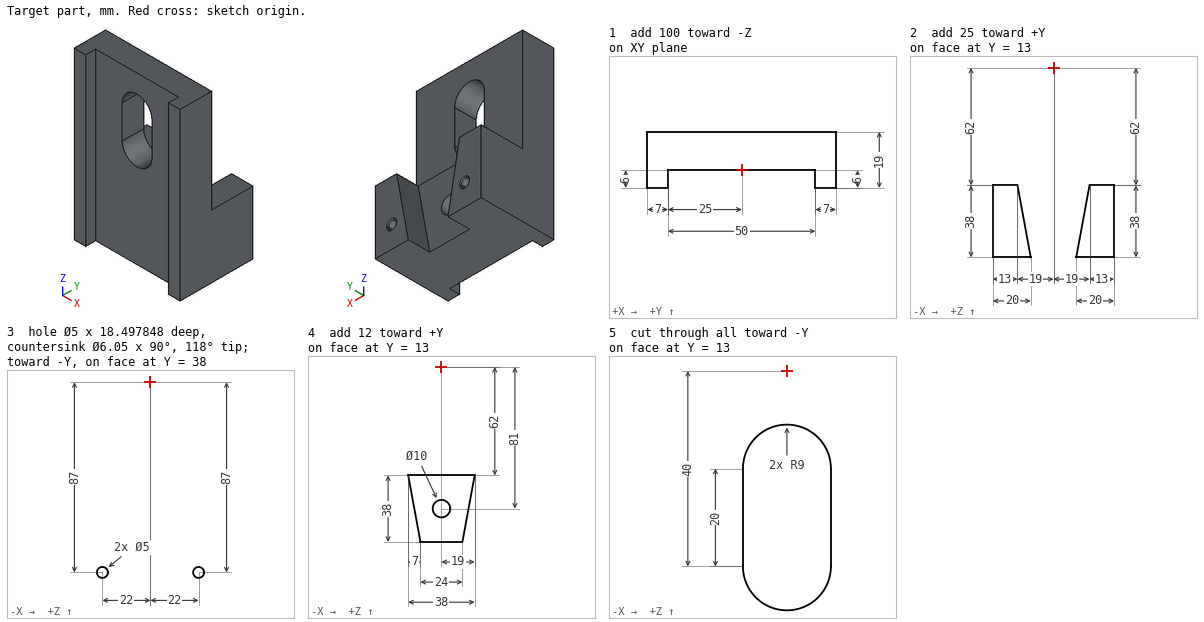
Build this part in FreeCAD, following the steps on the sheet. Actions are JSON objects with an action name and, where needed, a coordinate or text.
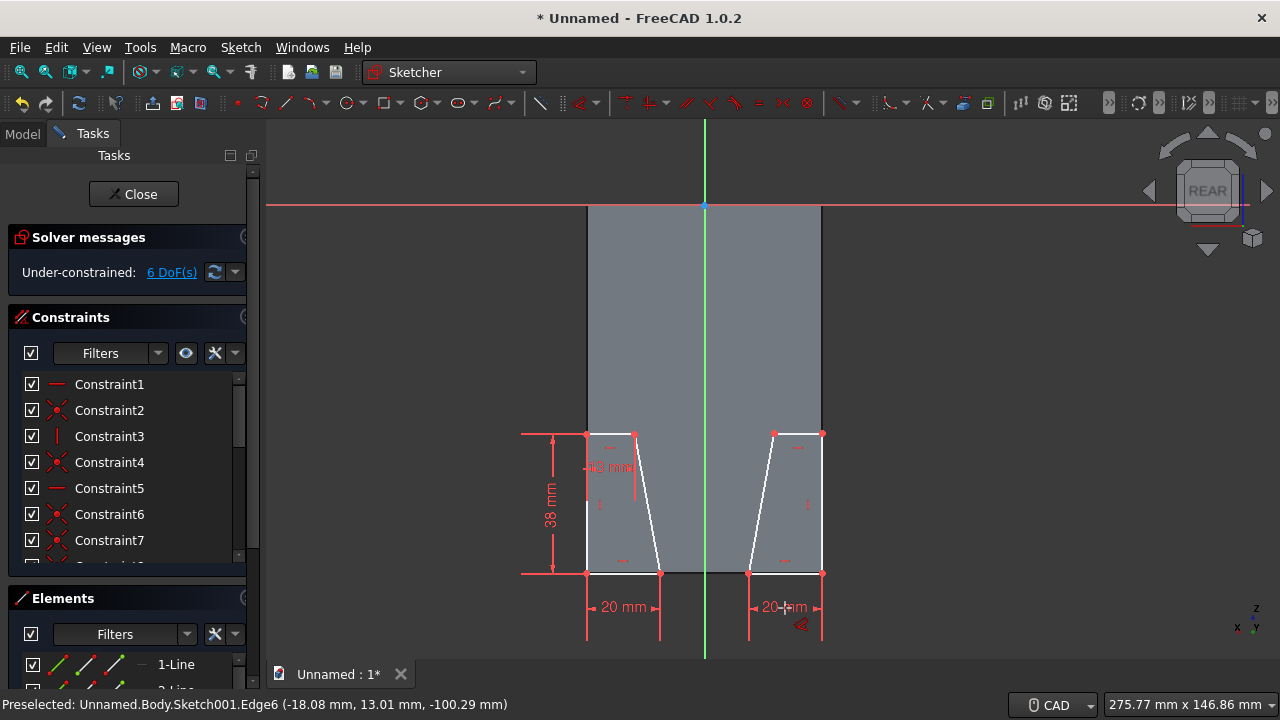
{"action": "left_click", "coordinate": [822, 532]}
{"action": "left_click", "coordinate": [856, 504]}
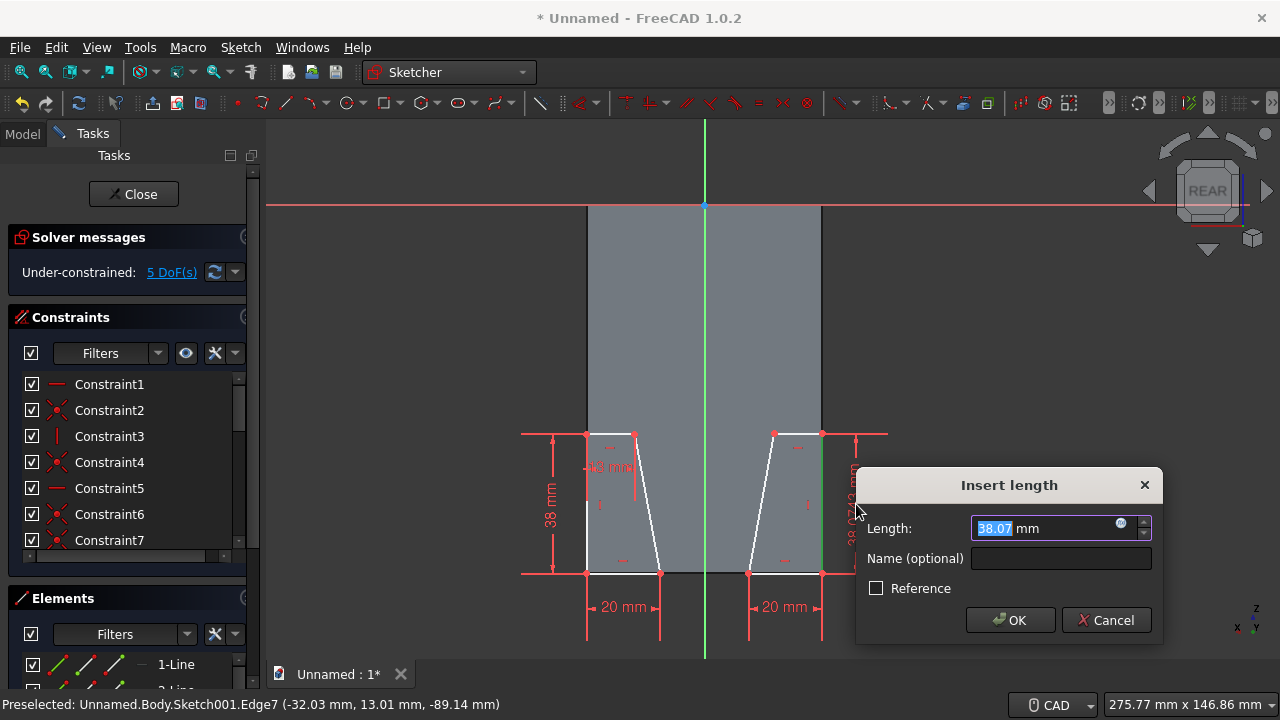
{"action": "type", "text": "38"}
{"action": "key", "text": "Return"}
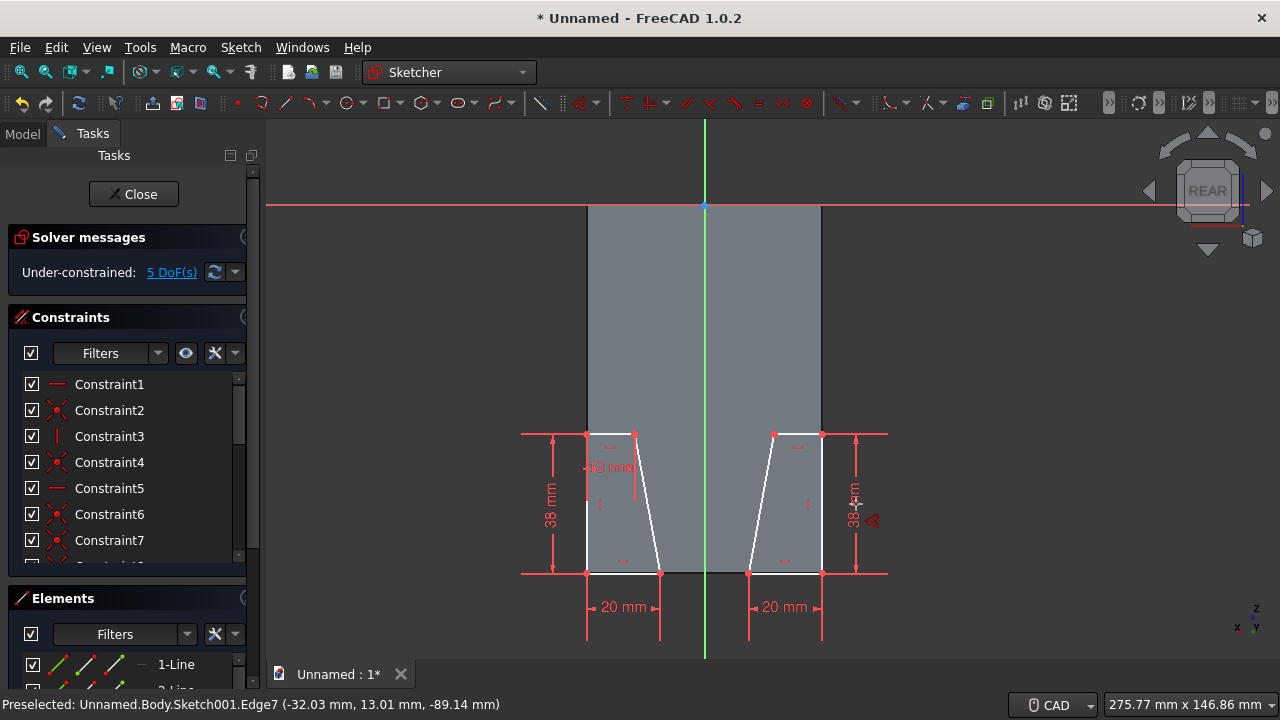
{"action": "left_click", "coordinate": [808, 434]}
{"action": "left_click", "coordinate": [798, 468]}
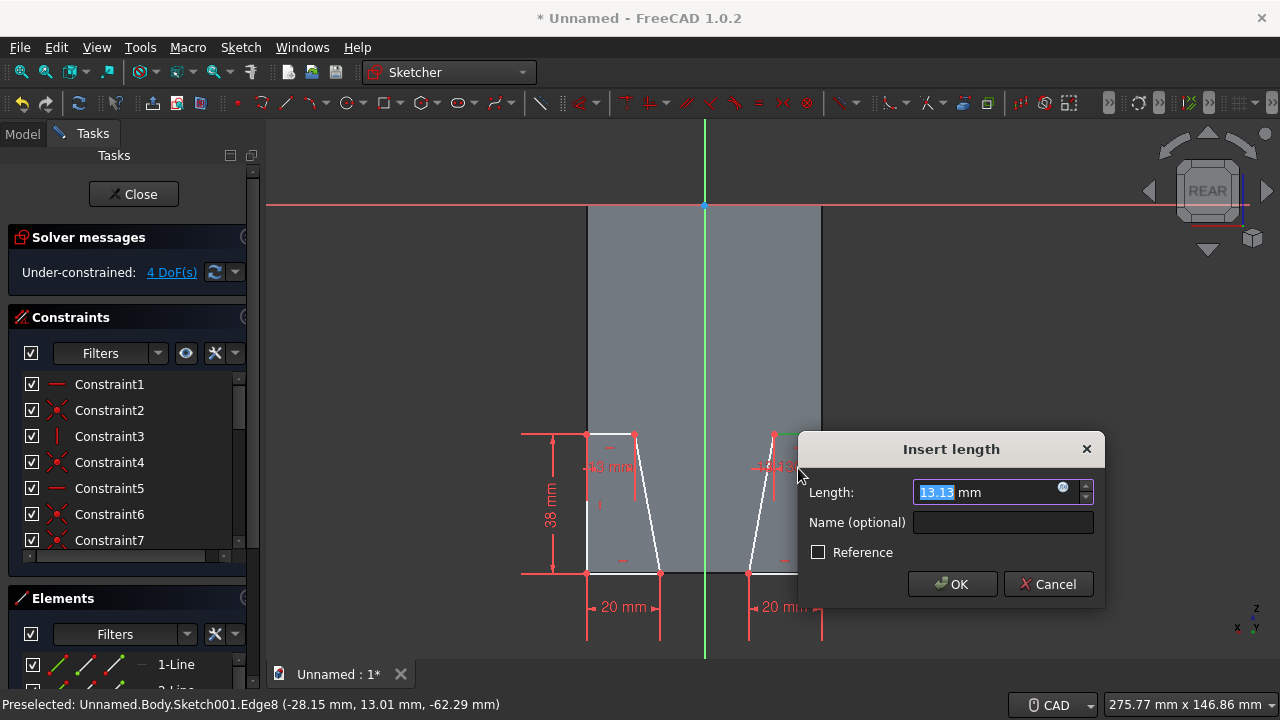
{"action": "type", "text": "13"}
{"action": "key", "text": "Return"}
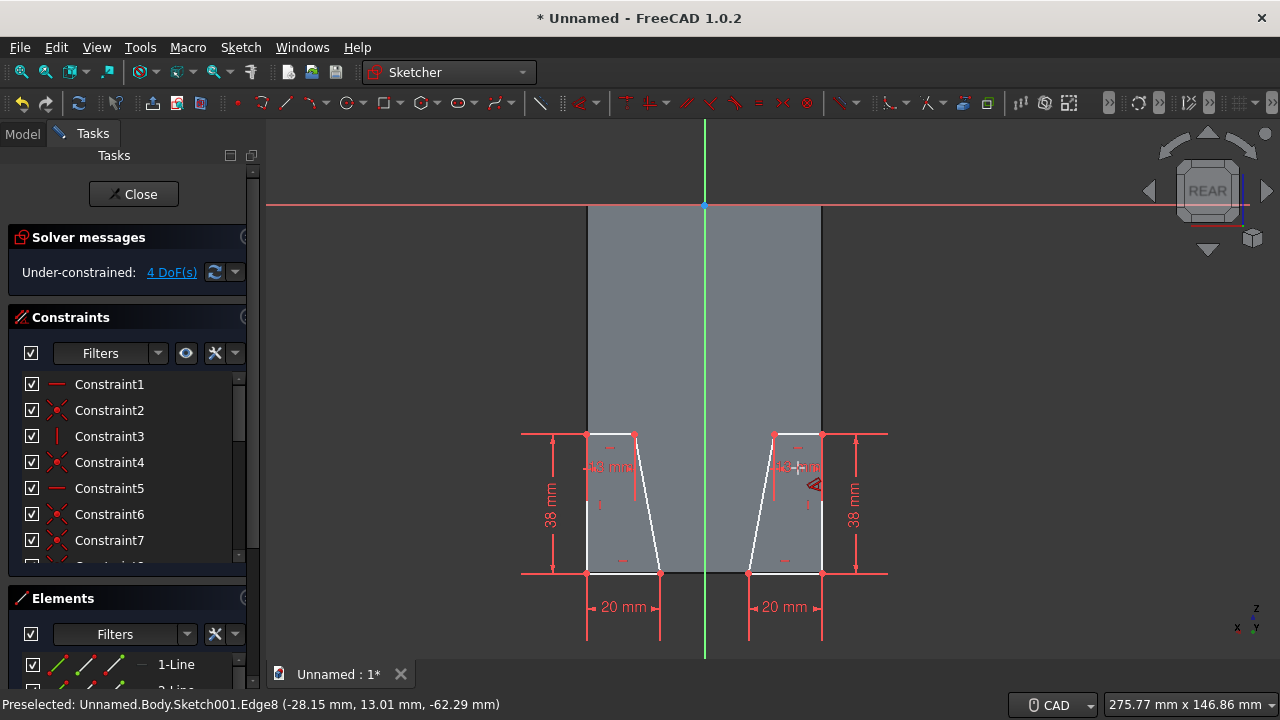
{"action": "left_click", "coordinate": [635, 434]}
{"action": "left_click", "coordinate": [670, 171]}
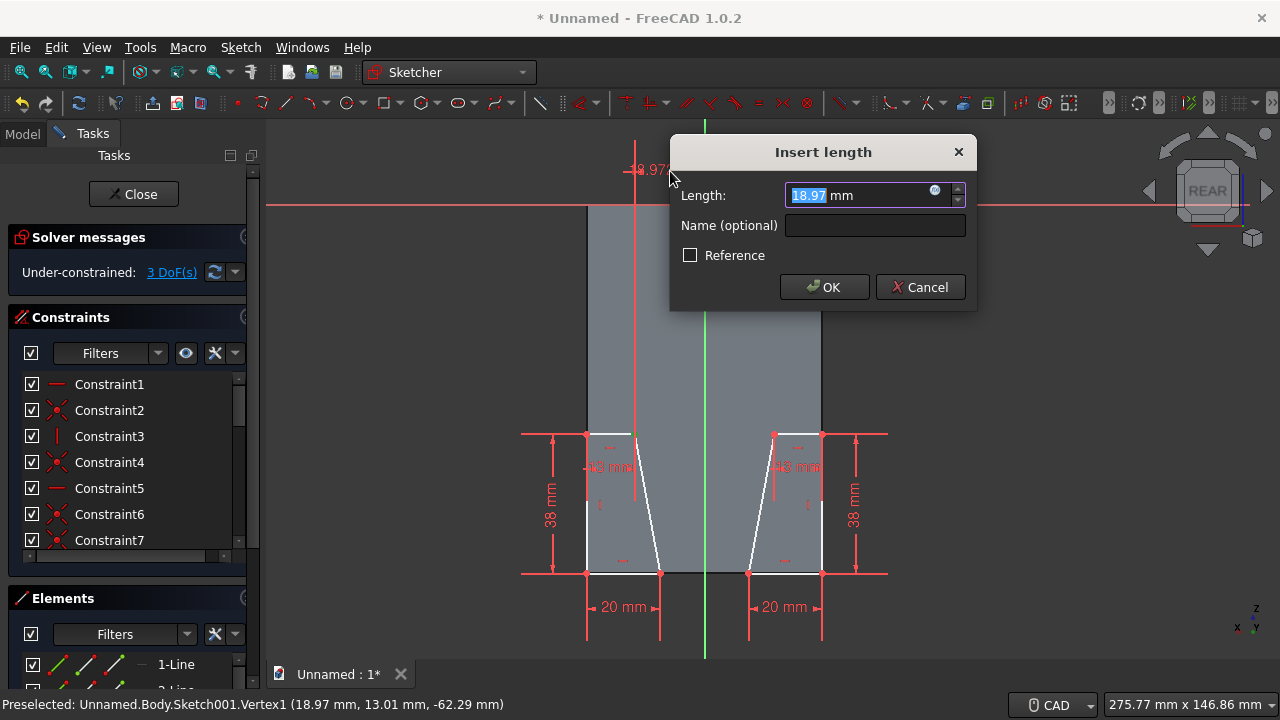
{"action": "type", "text": "19"}
{"action": "key", "text": "Return"}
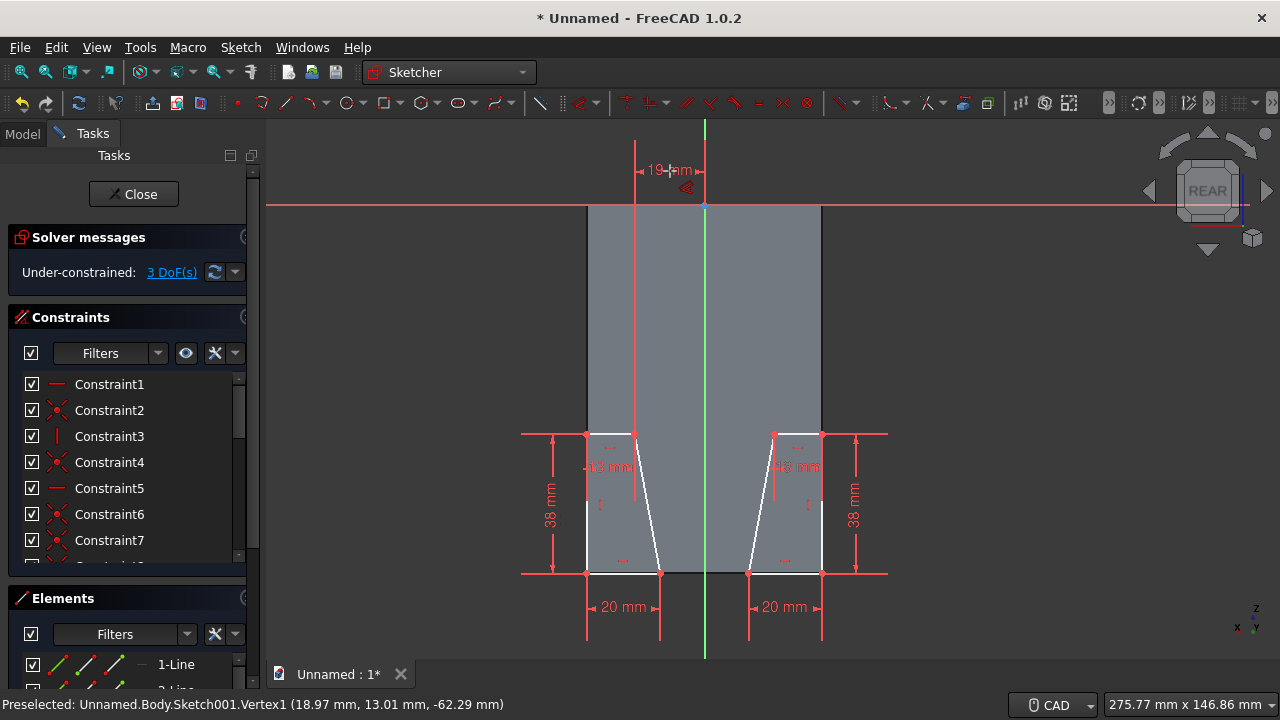
{"action": "left_click", "coordinate": [635, 434]}
{"action": "left_click", "coordinate": [601, 320]}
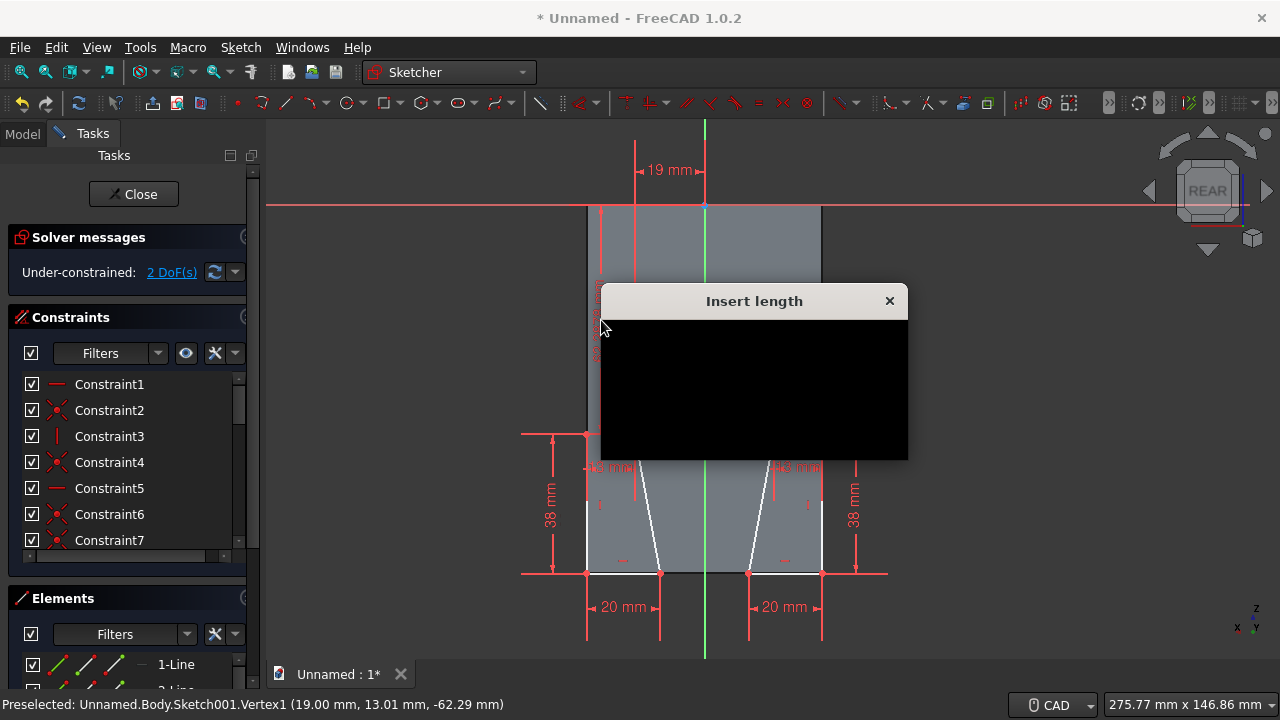
{"action": "type", "text": "62"}
{"action": "key", "text": "Return"}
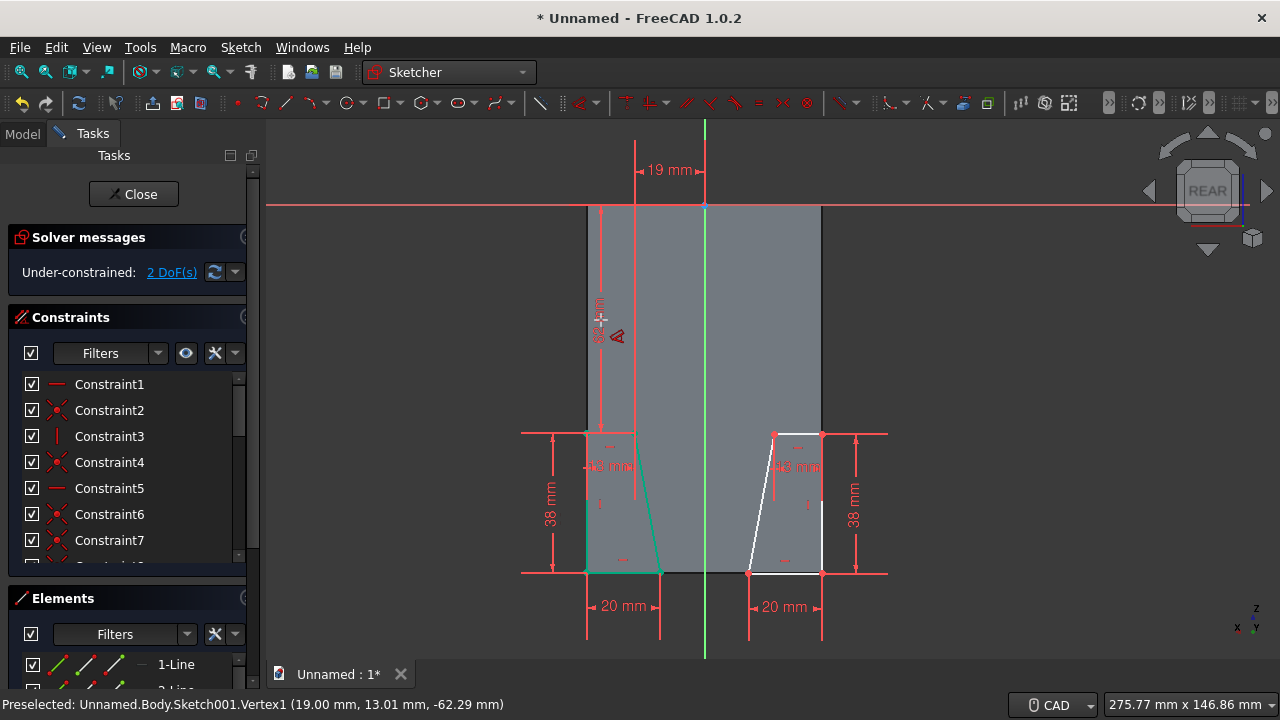
{"action": "left_click", "coordinate": [774, 434]}
{"action": "left_click", "coordinate": [756, 171]}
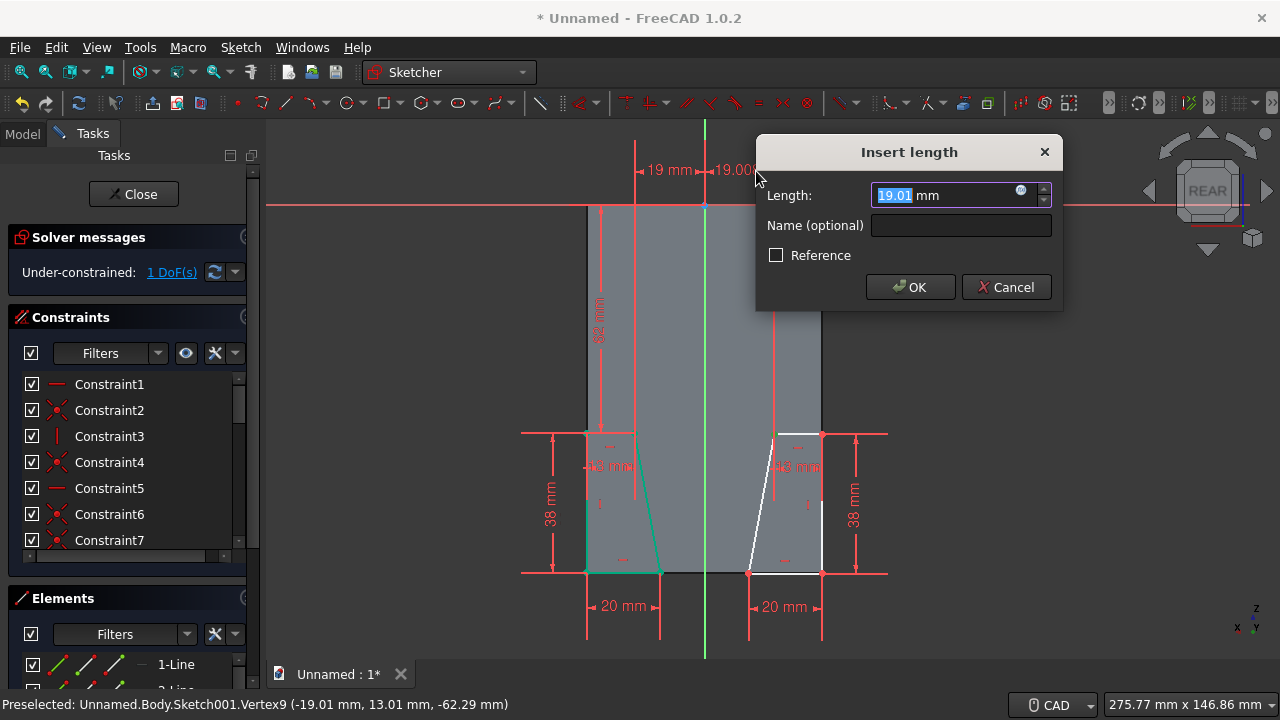
{"action": "type", "text": "19"}
{"action": "key", "text": "Return"}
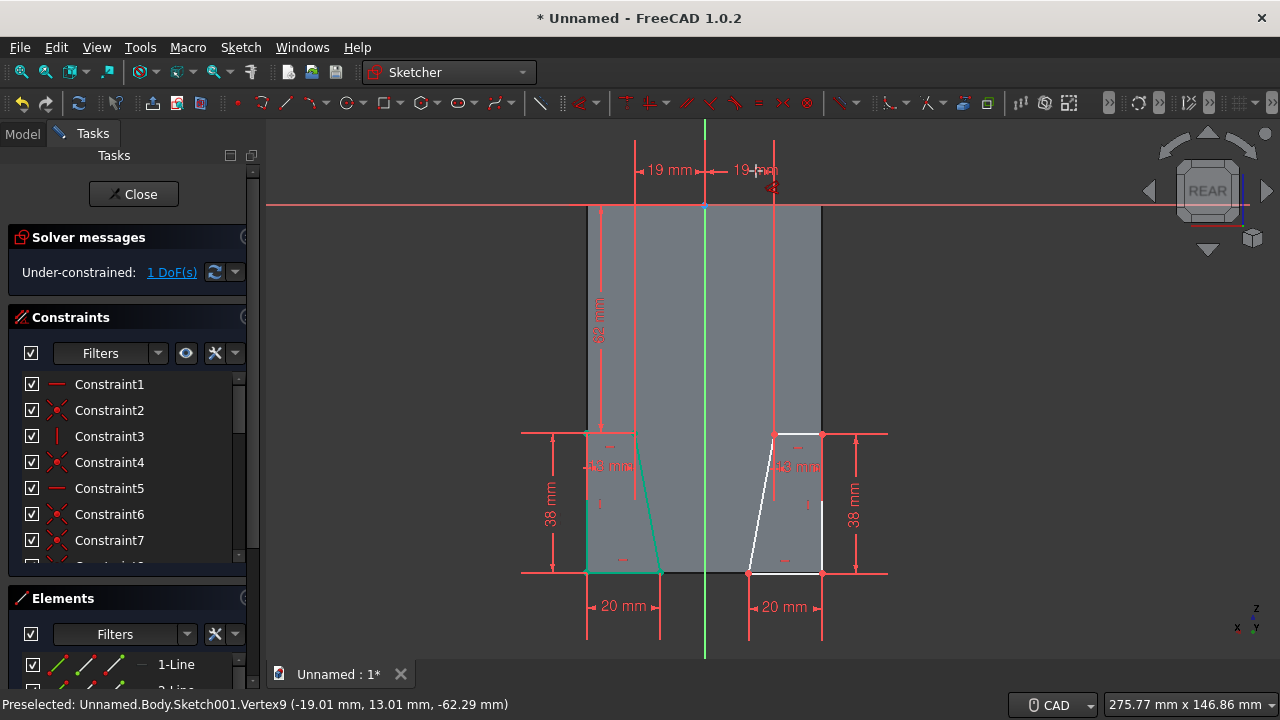
{"action": "left_click", "coordinate": [774, 434]}
{"action": "left_click", "coordinate": [808, 320]}